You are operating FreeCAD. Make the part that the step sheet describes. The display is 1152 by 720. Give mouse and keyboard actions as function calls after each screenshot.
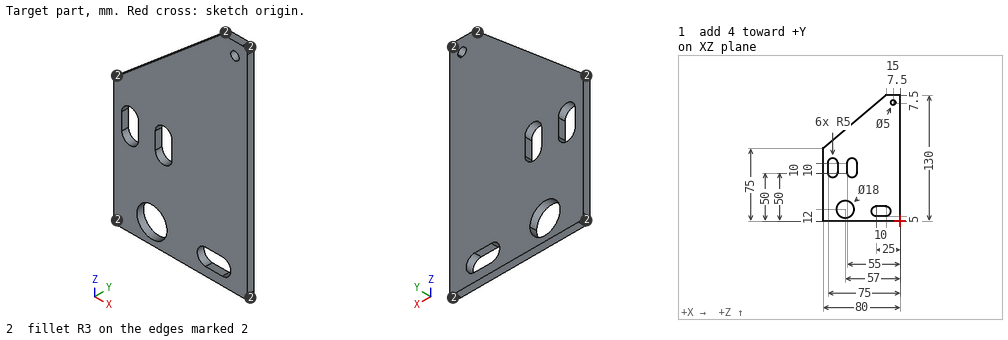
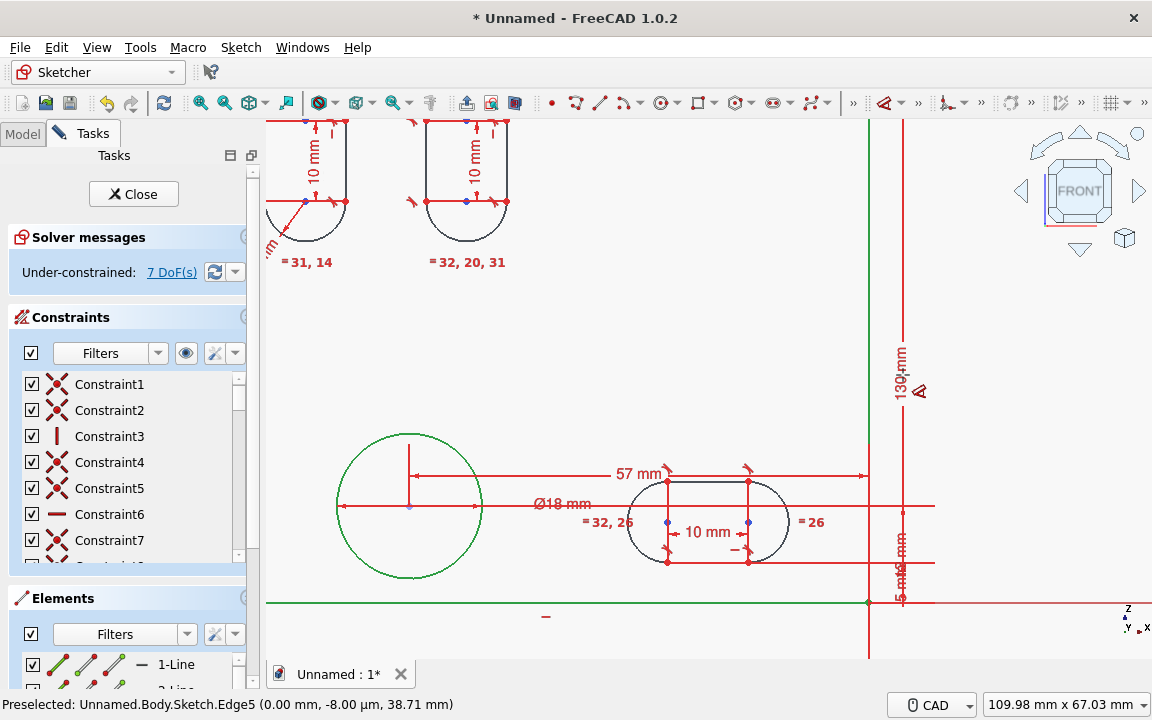
scroll(681, 523, down, 6)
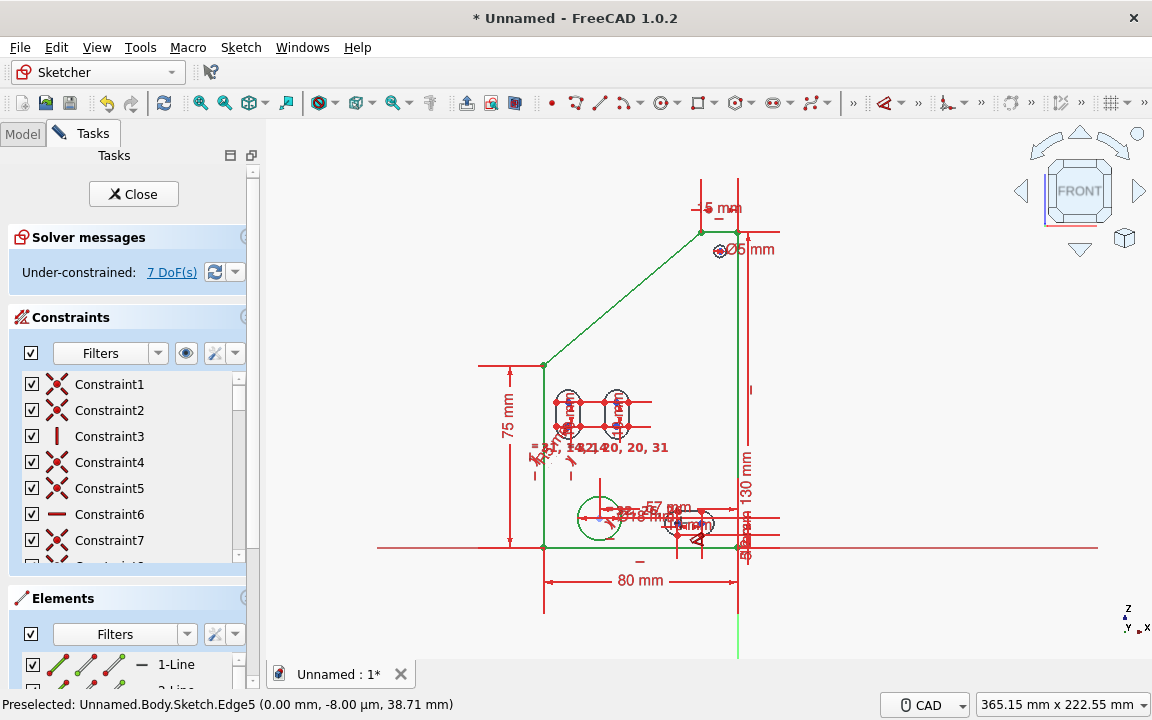
click(556, 427)
click(647, 393)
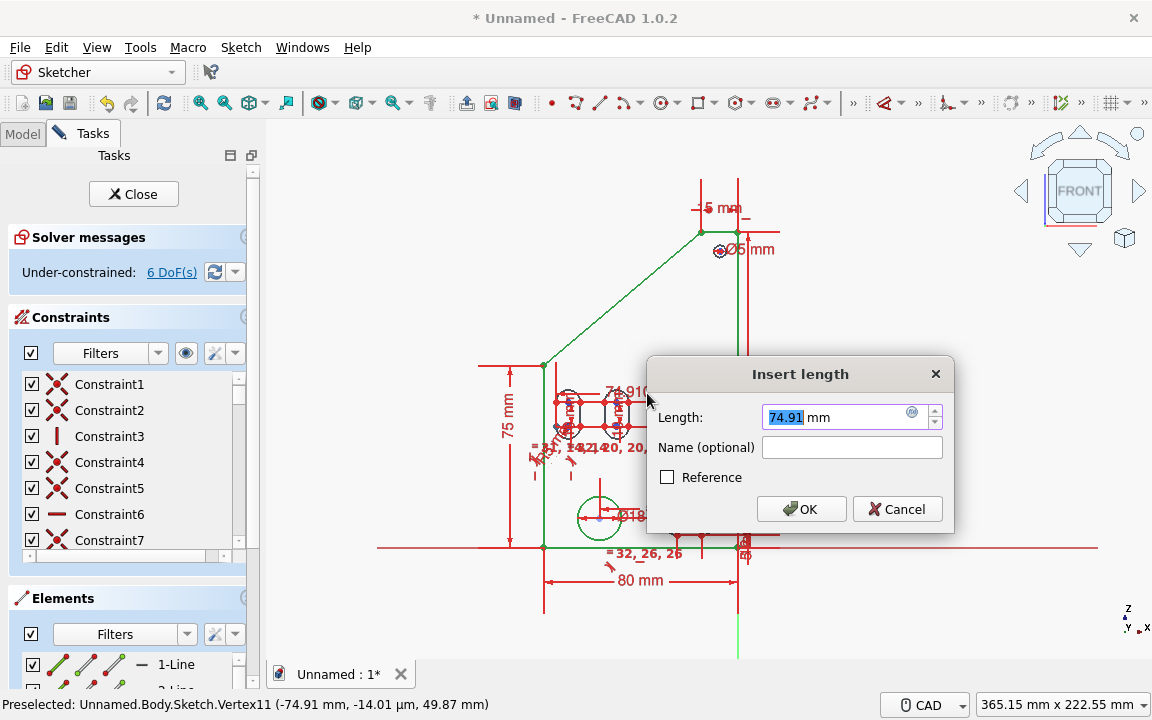
text(75)
key(Return)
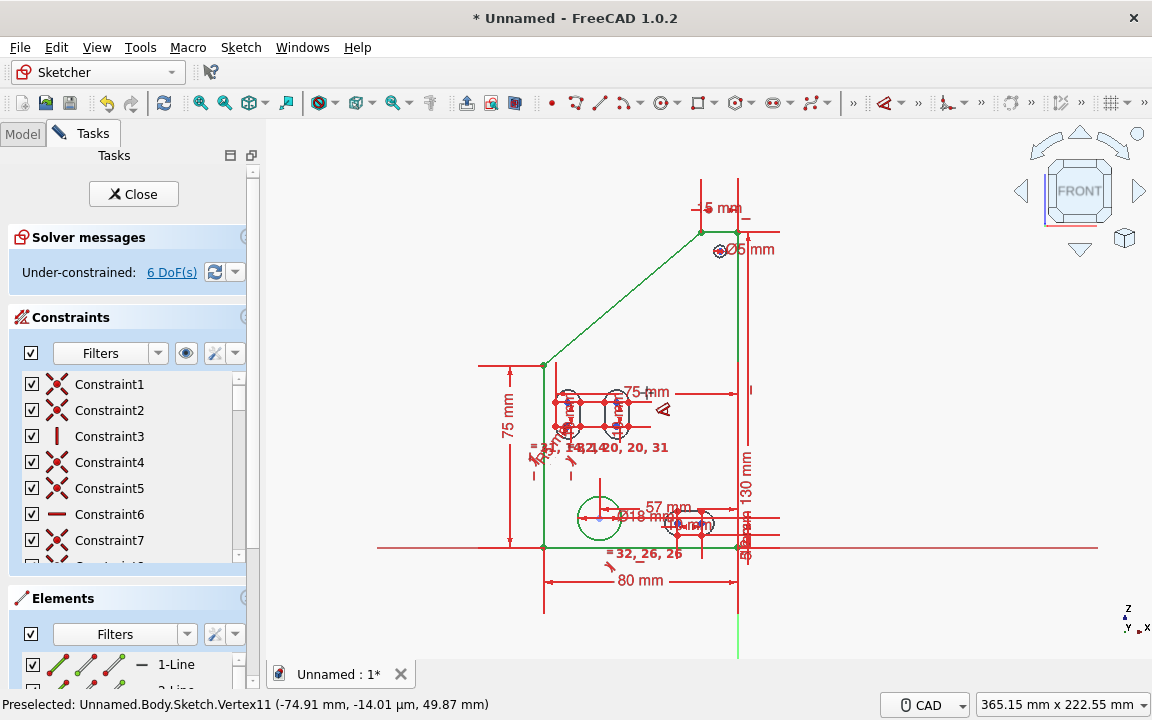
click(556, 427)
click(772, 445)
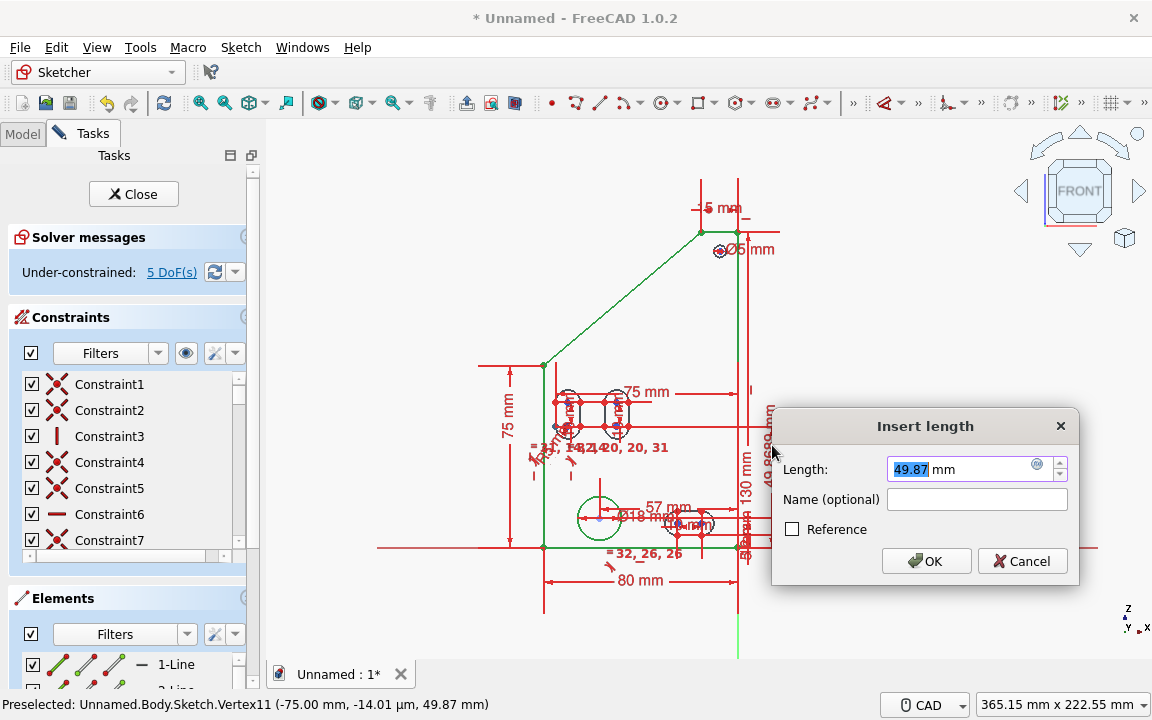
text(50)
key(Return)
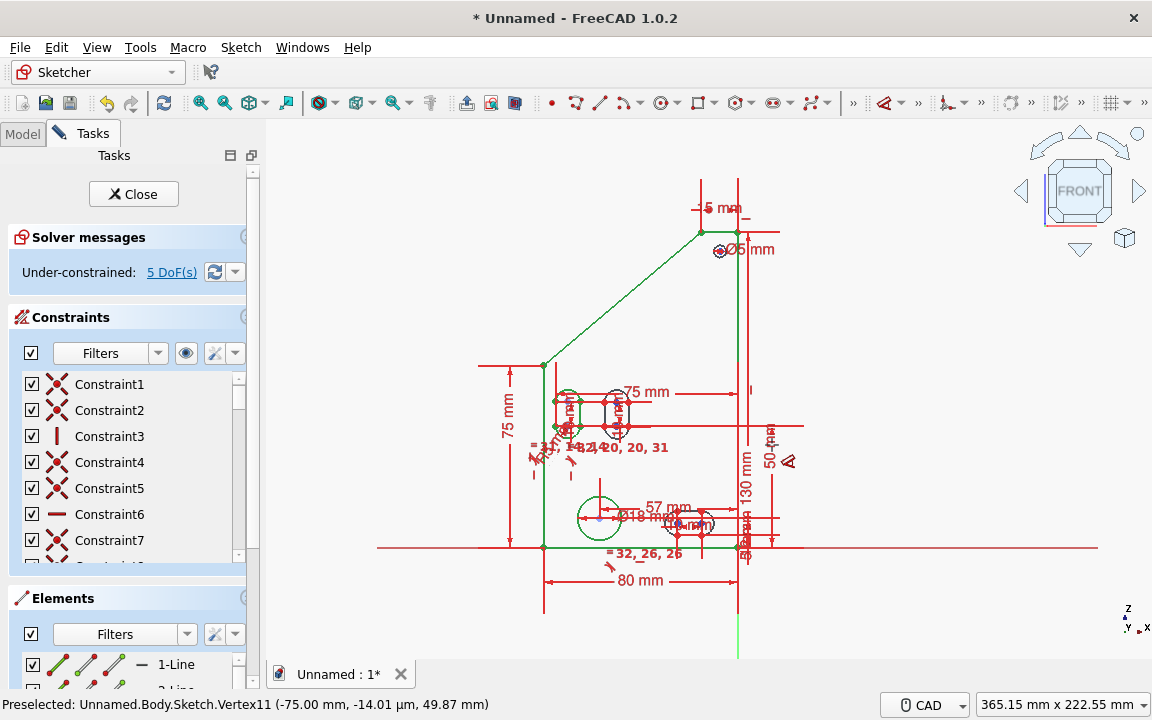
click(605, 427)
click(718, 582)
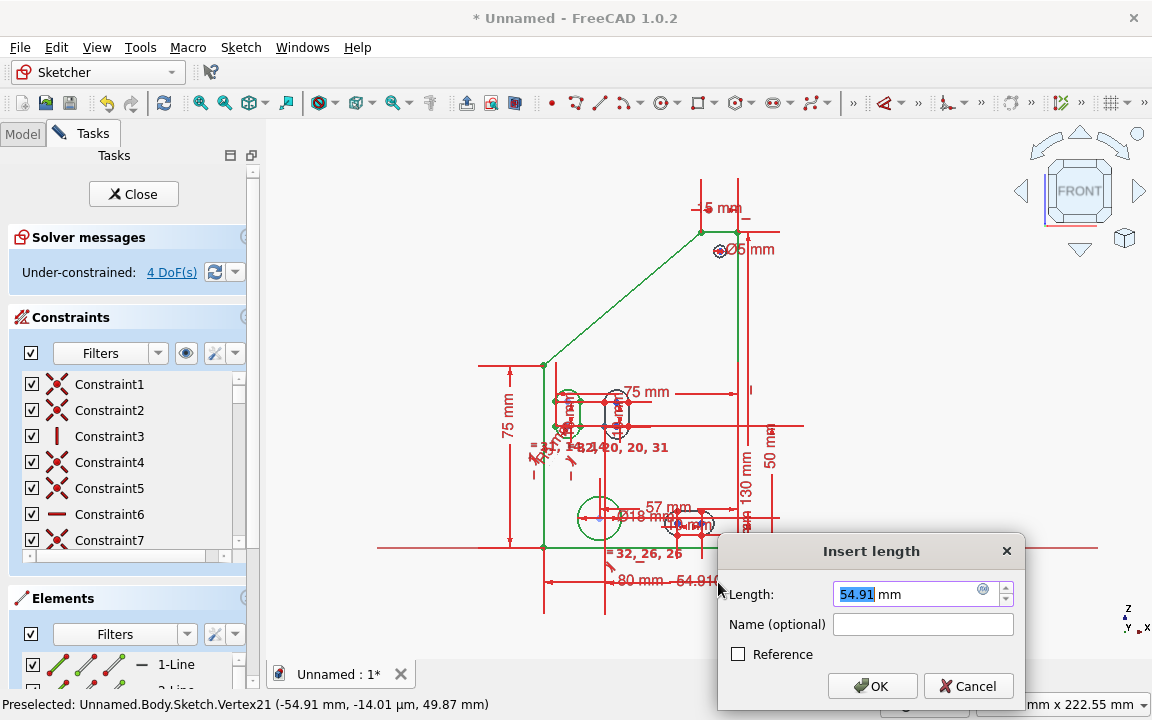
text(55)
key(Return)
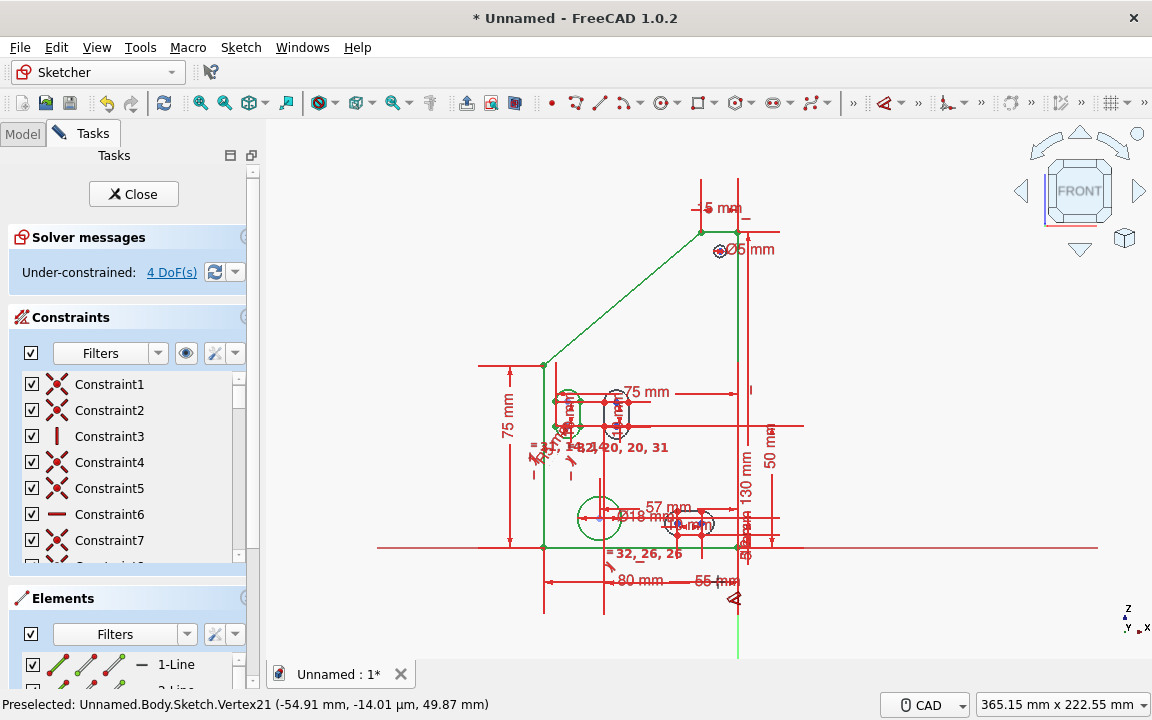
click(604, 427)
click(570, 487)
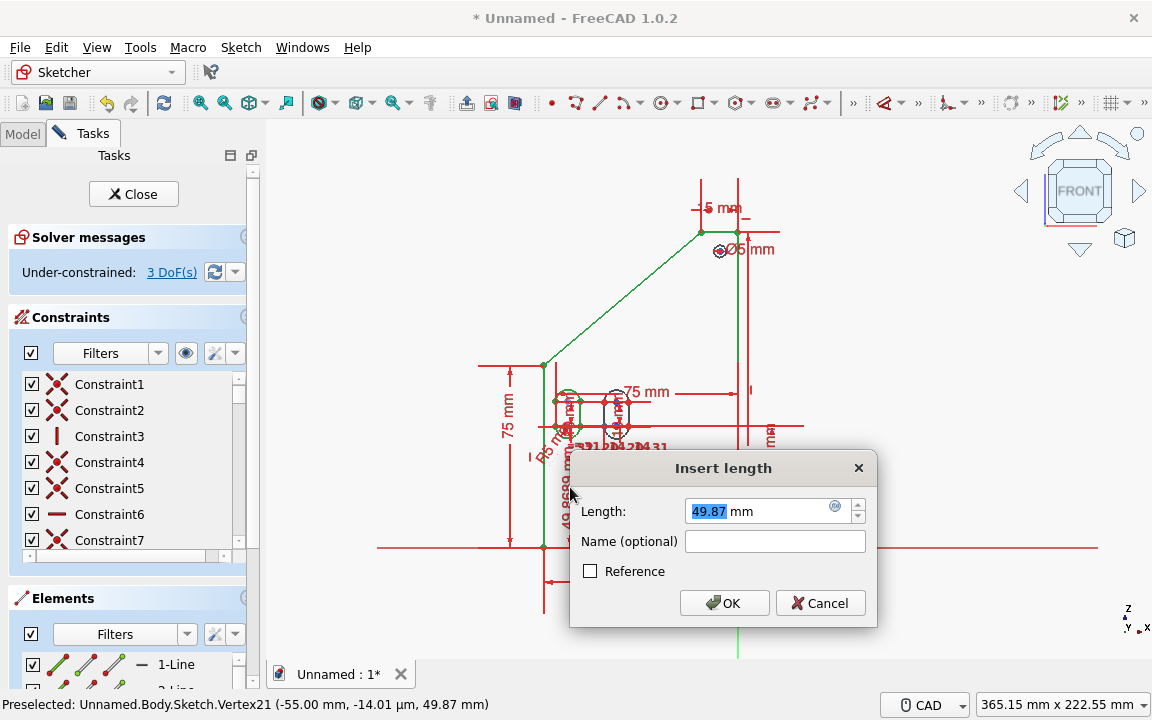
text(50)
key(Return)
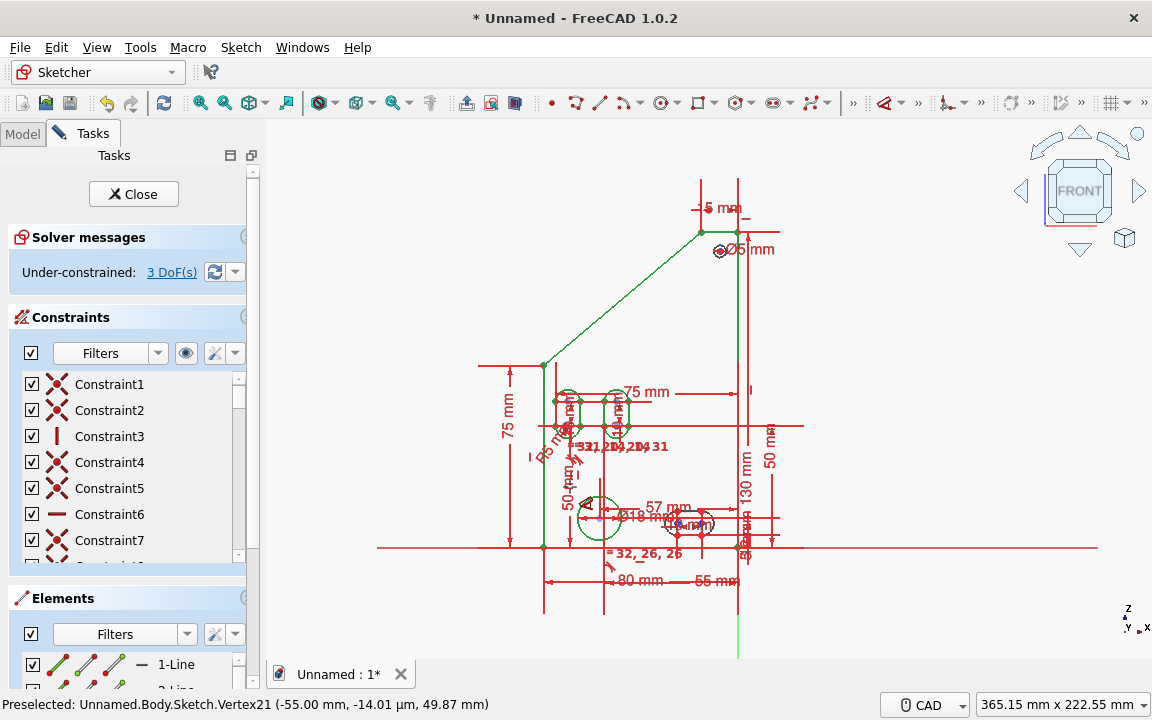
click(677, 511)
click(708, 606)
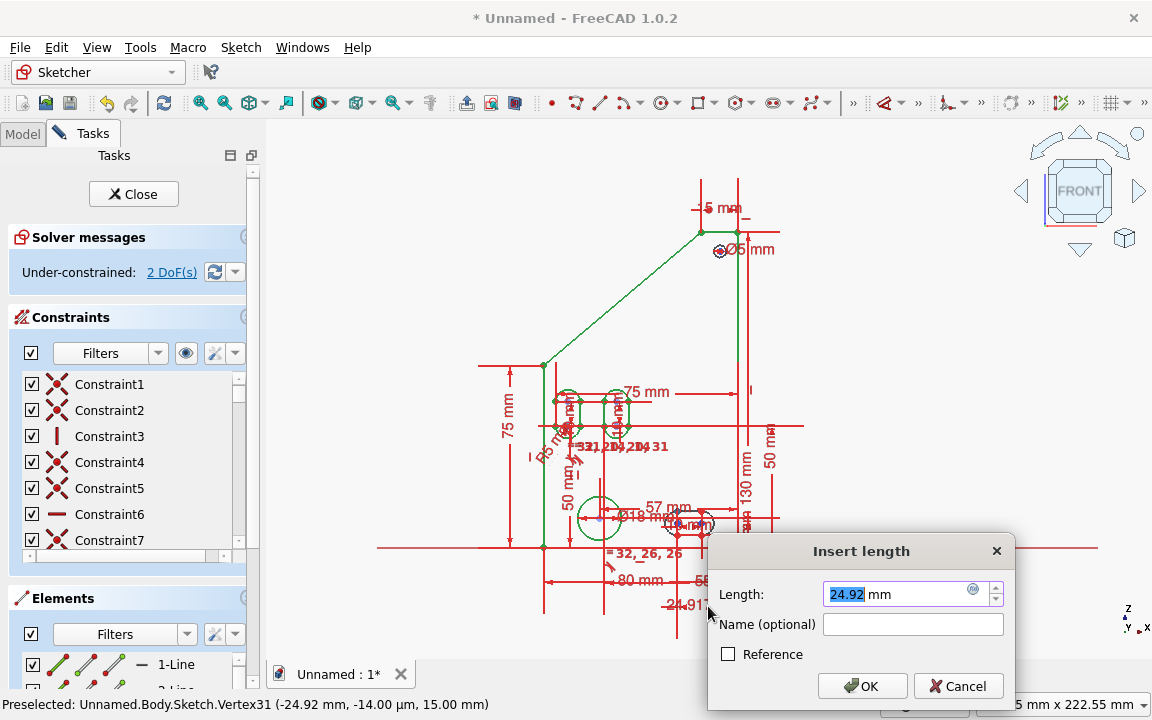
text(25)
key(Return)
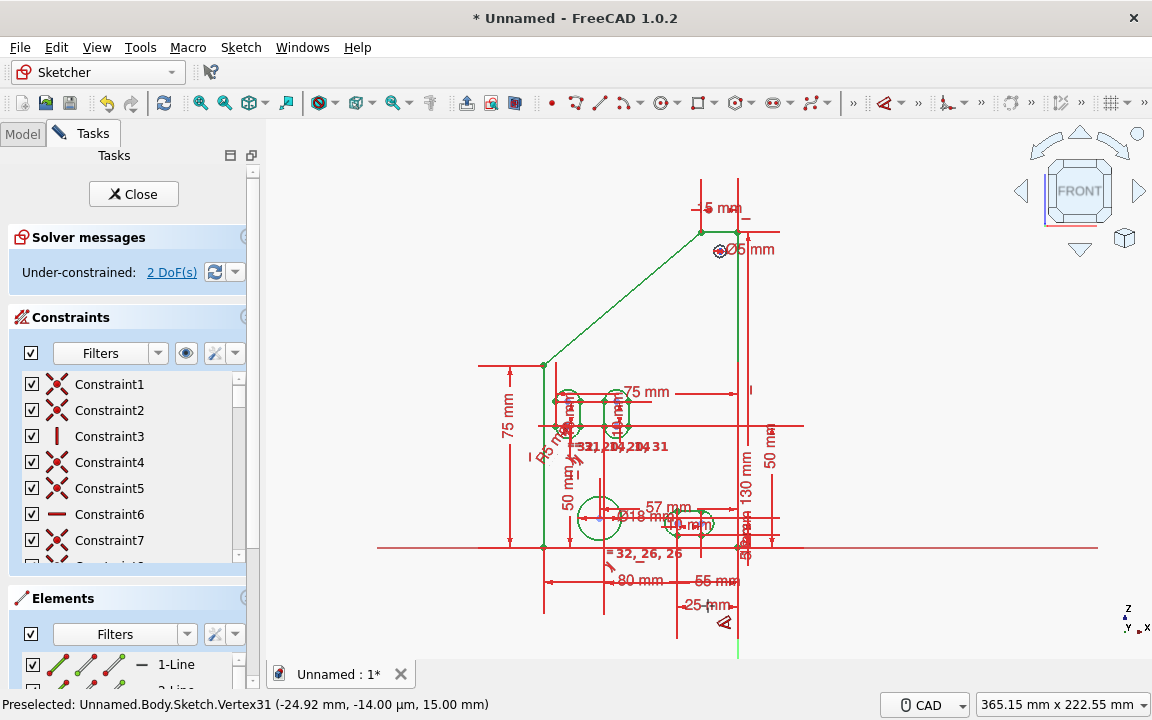
scroll(720, 251, up, 4)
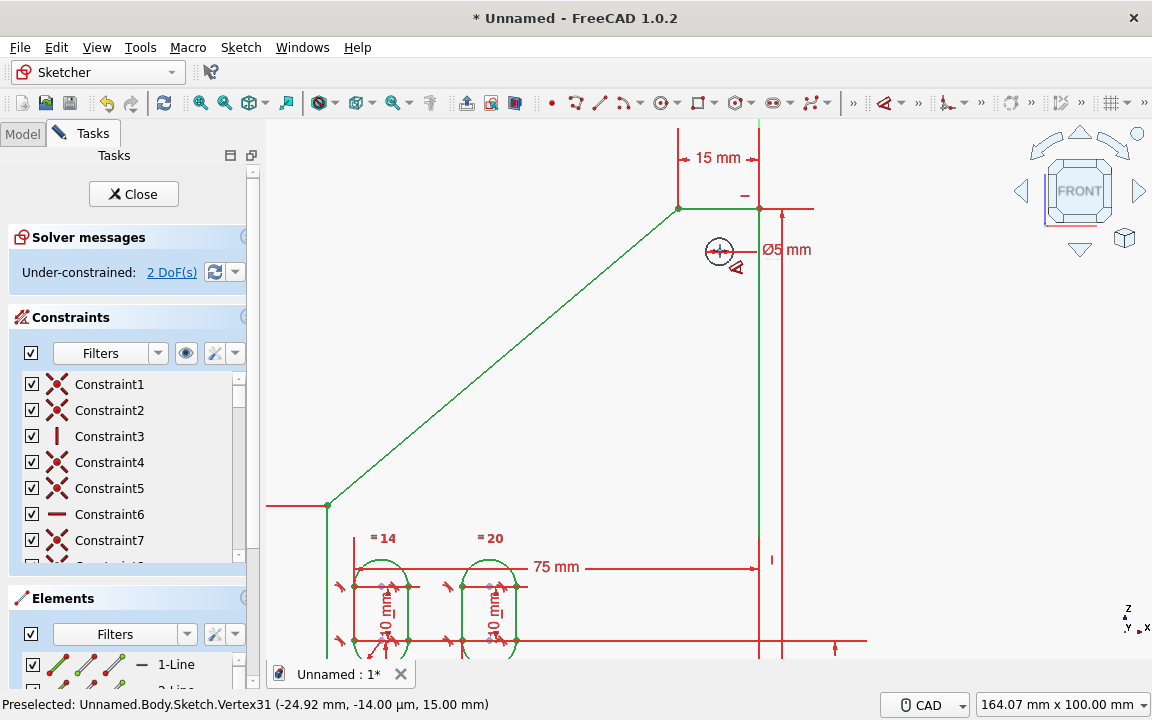
click(719, 252)
click(739, 194)